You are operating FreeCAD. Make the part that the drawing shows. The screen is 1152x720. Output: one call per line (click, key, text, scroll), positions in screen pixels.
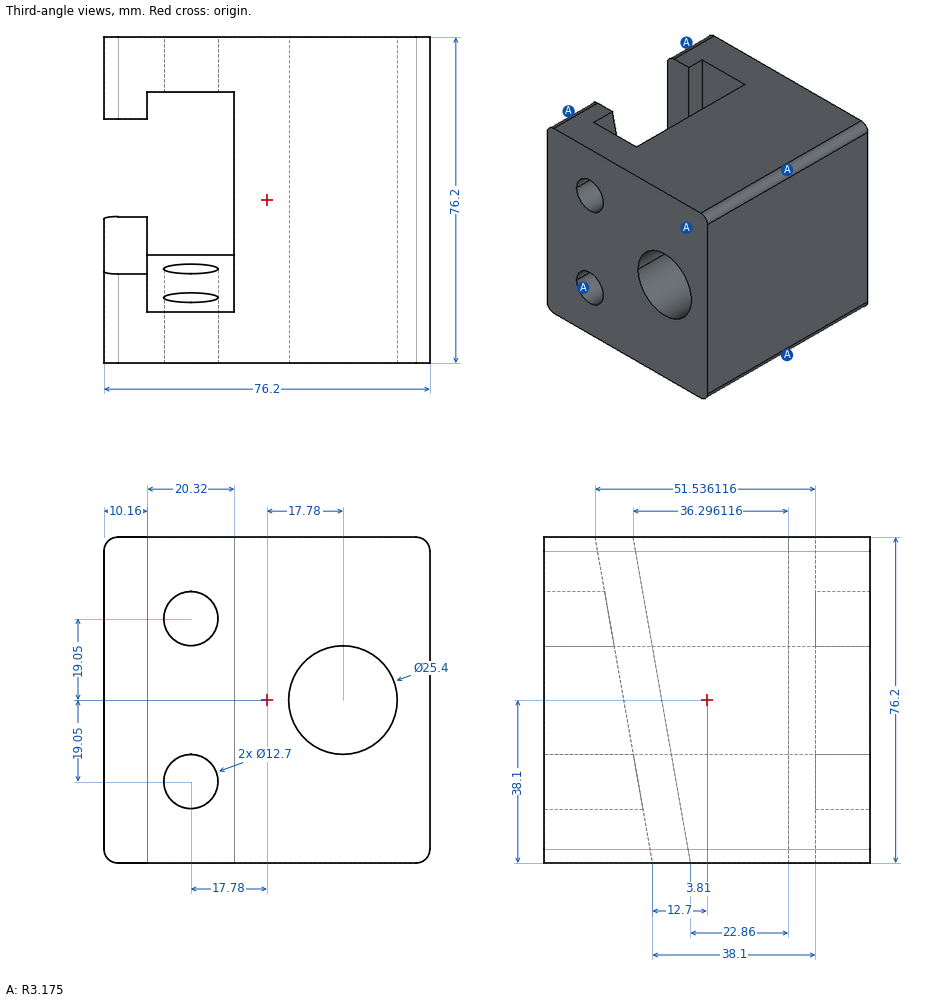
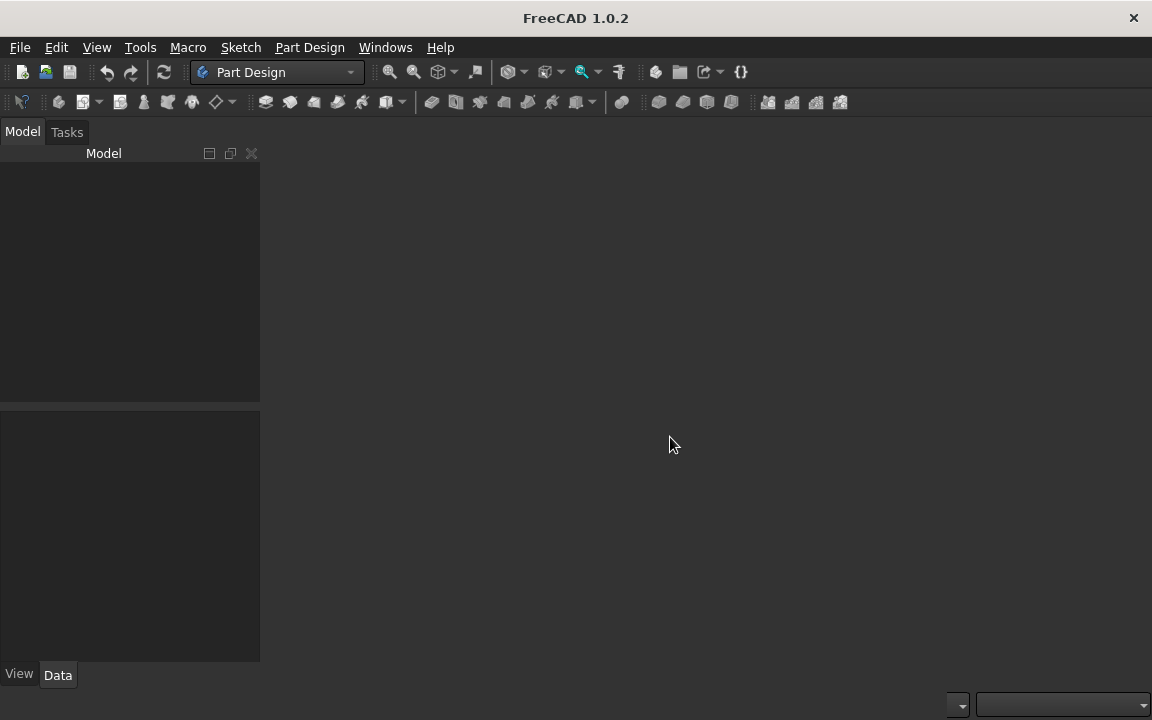
key(ctrl+n)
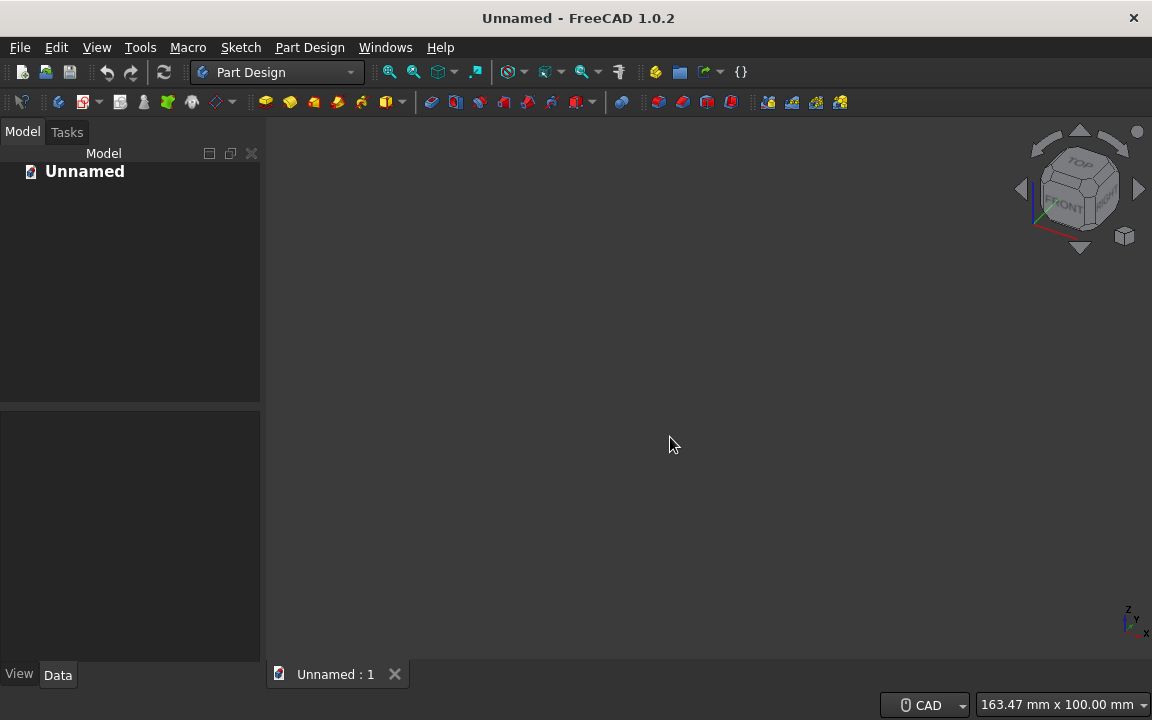
click(84, 102)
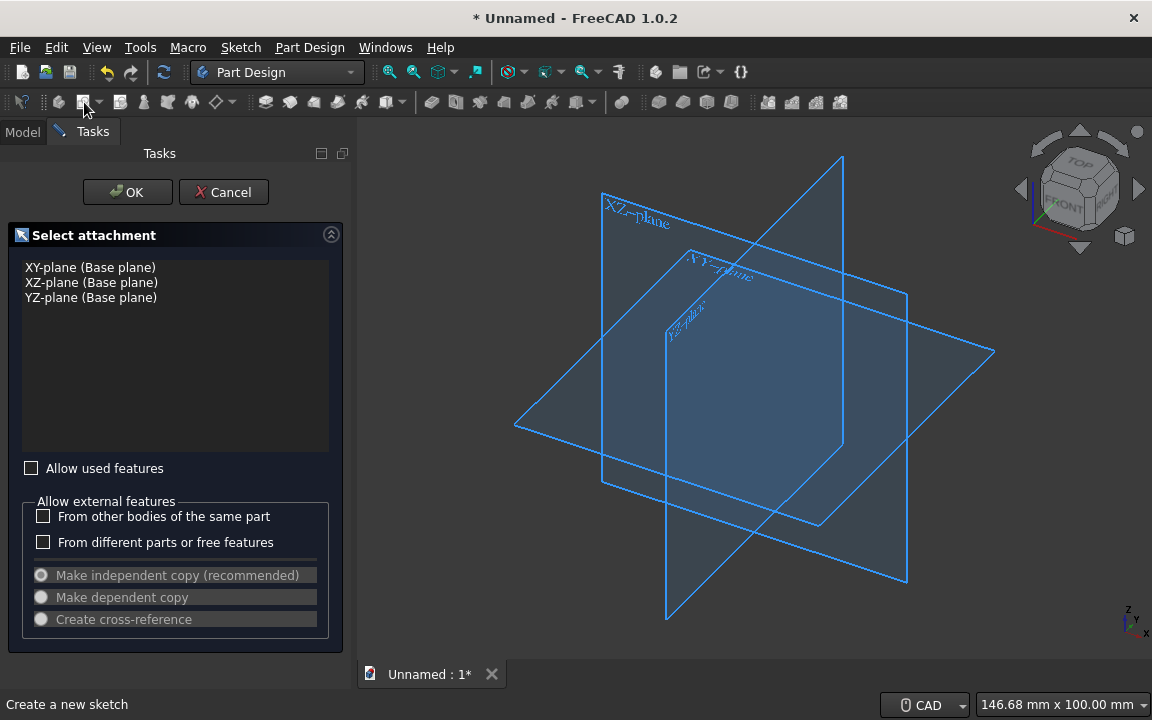
click(82, 268)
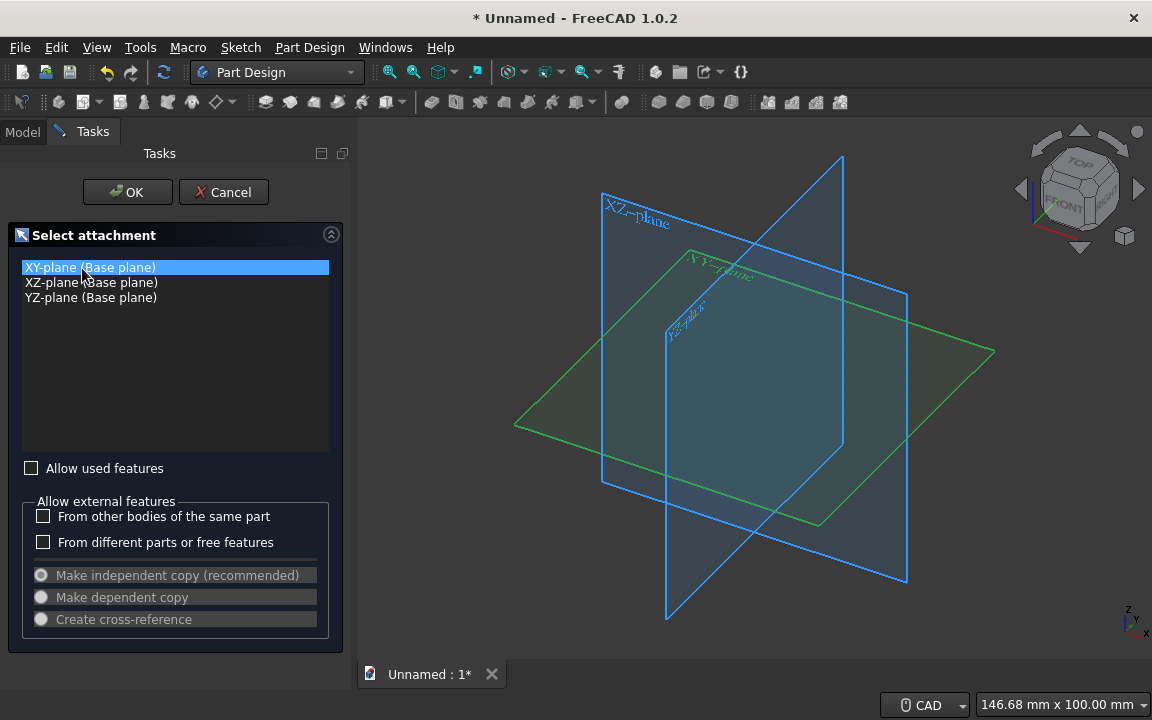
click(128, 192)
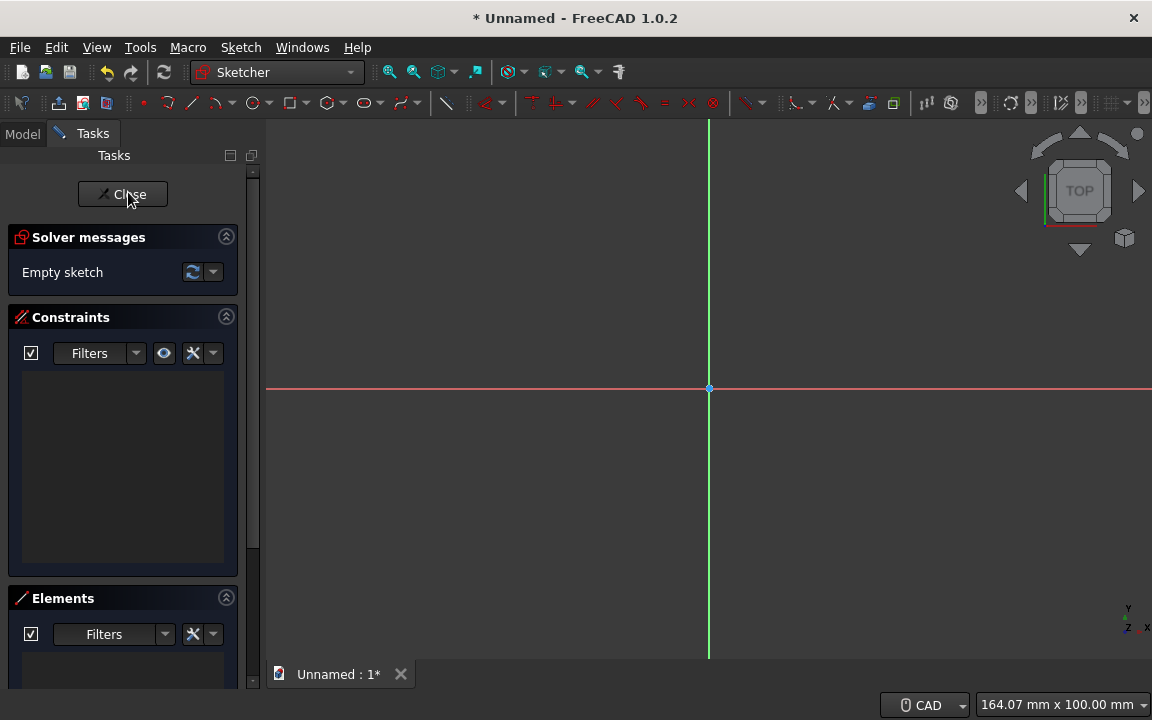
key(g)
key(v)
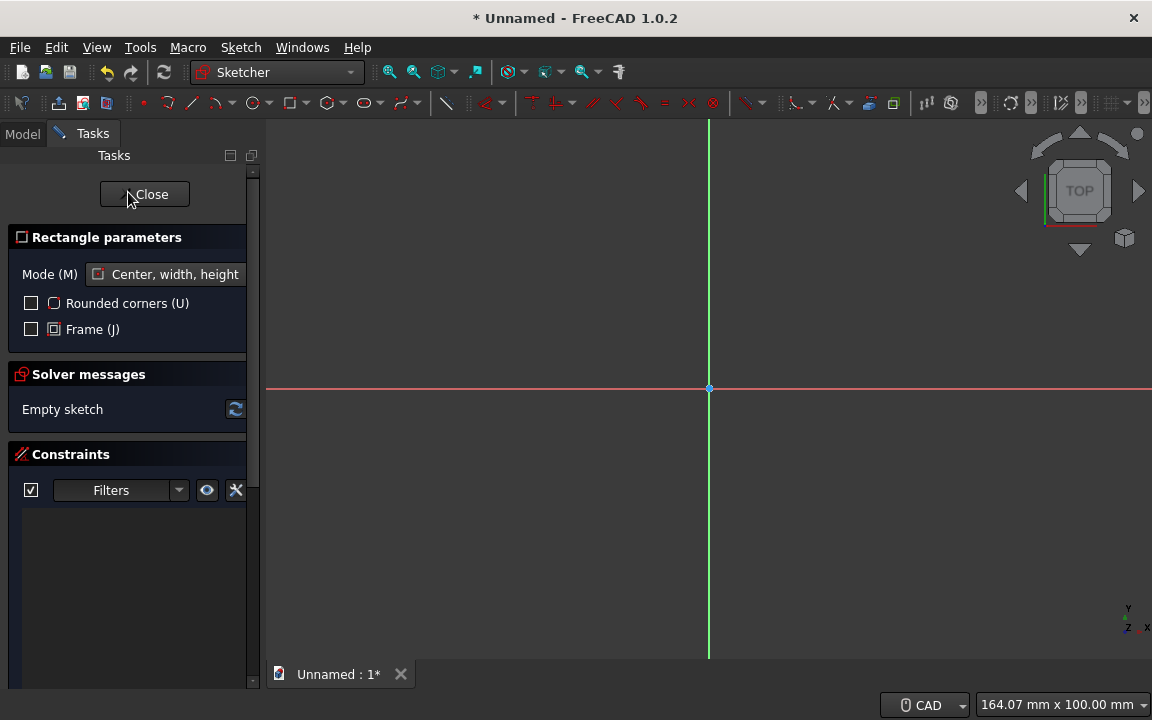
click(709, 389)
click(915, 183)
key(Escape)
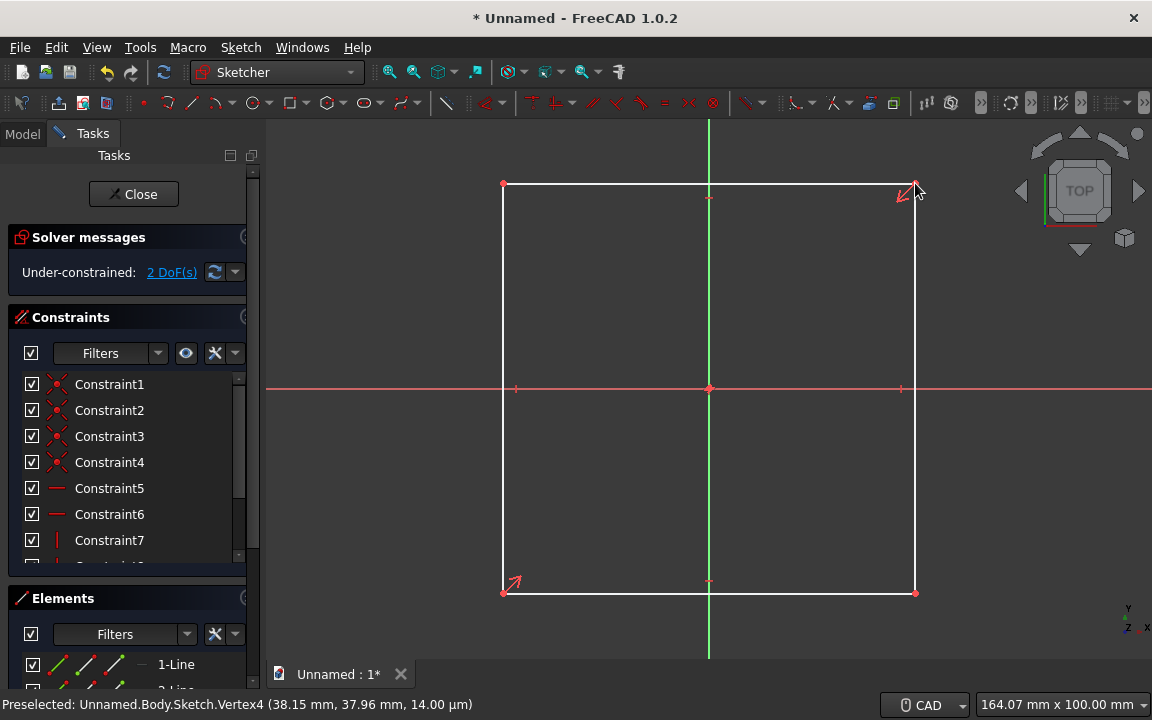
key(d)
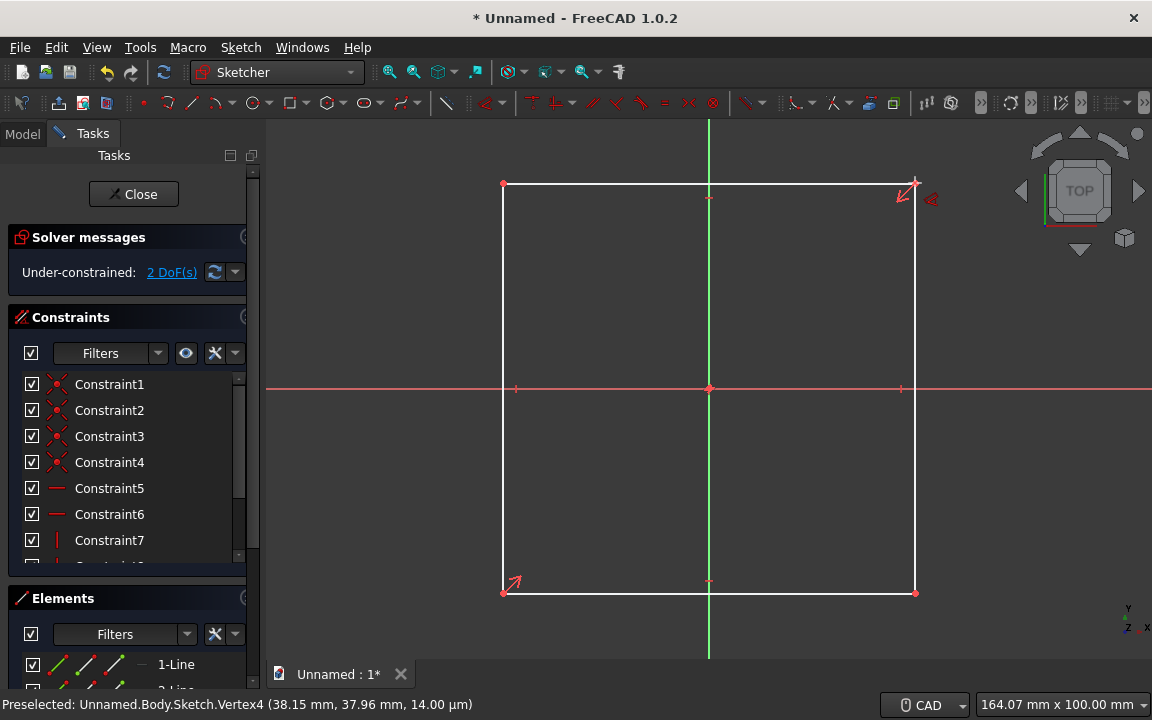
click(627, 594)
click(614, 628)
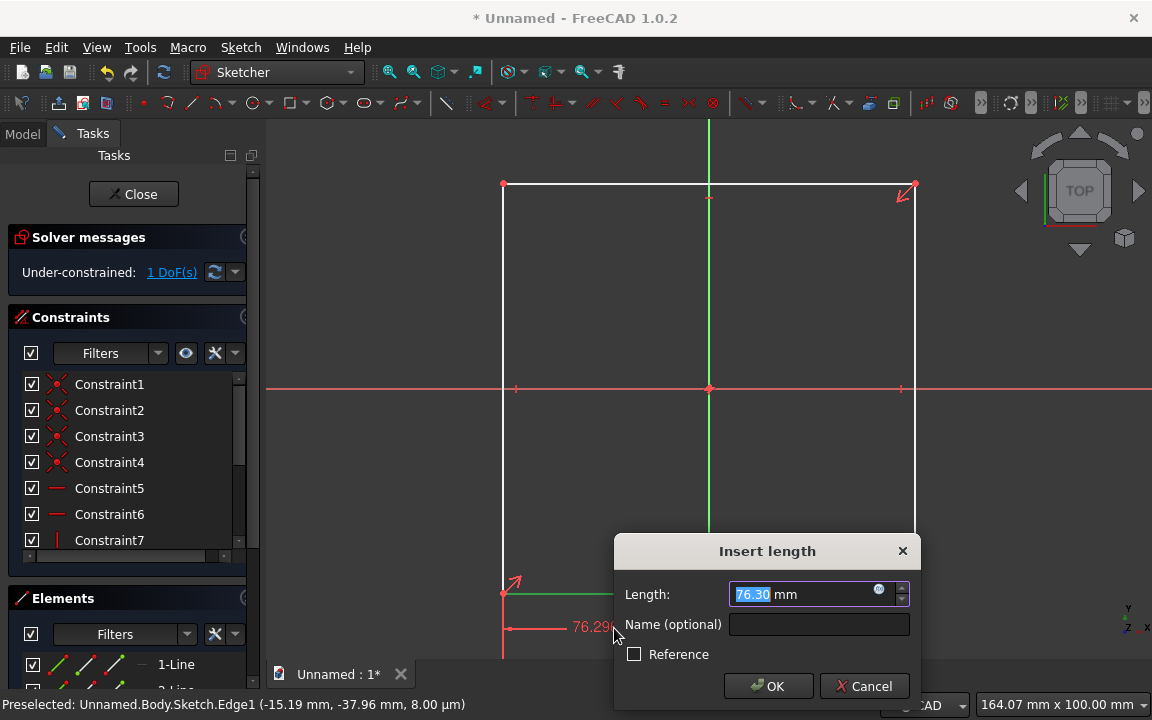
text(76.2)
key(Return)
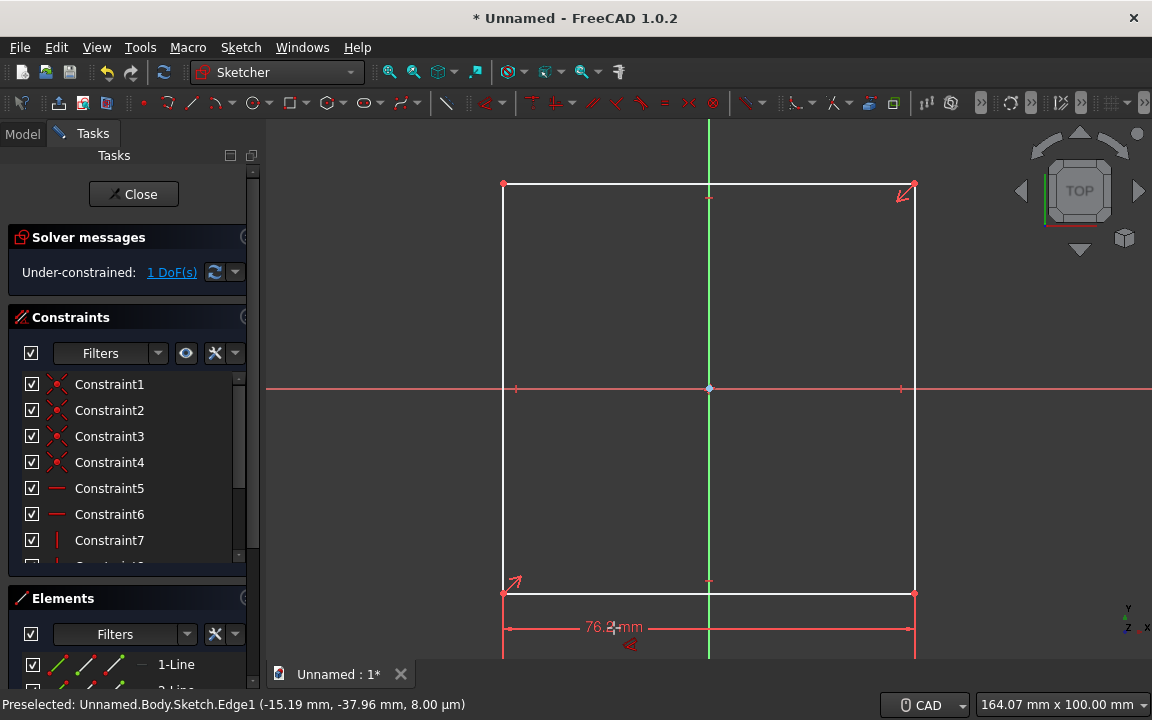
click(915, 471)
click(949, 295)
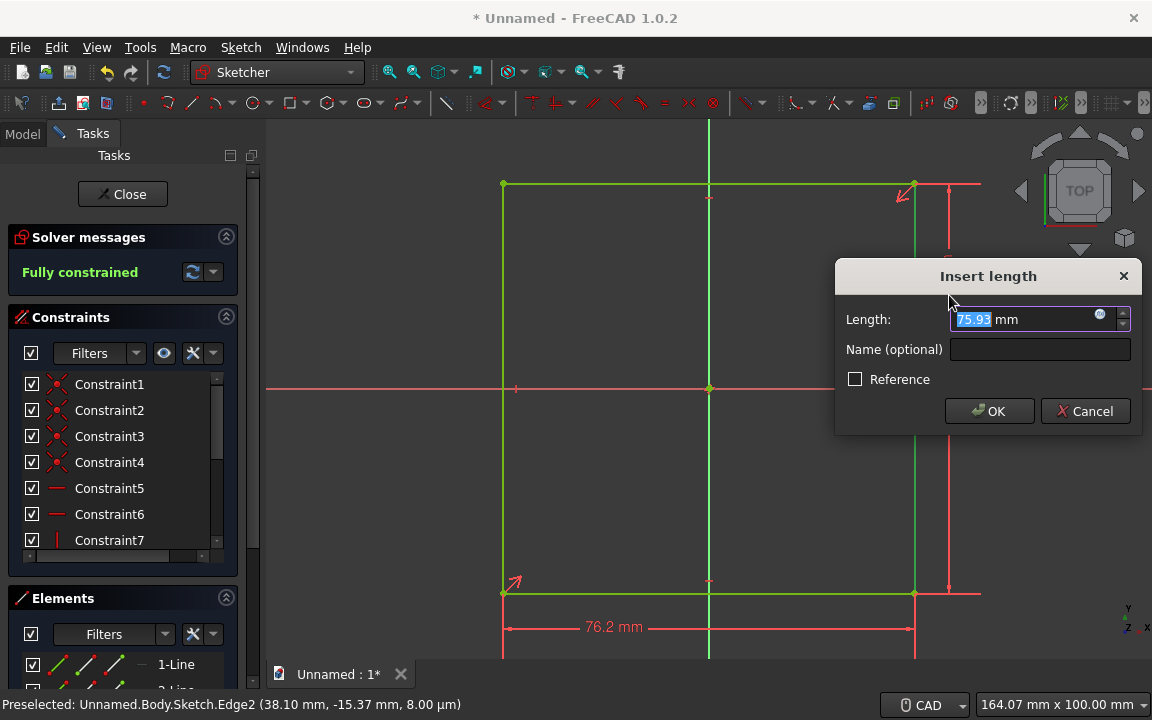
text(76.2)
key(Return)
key(Escape)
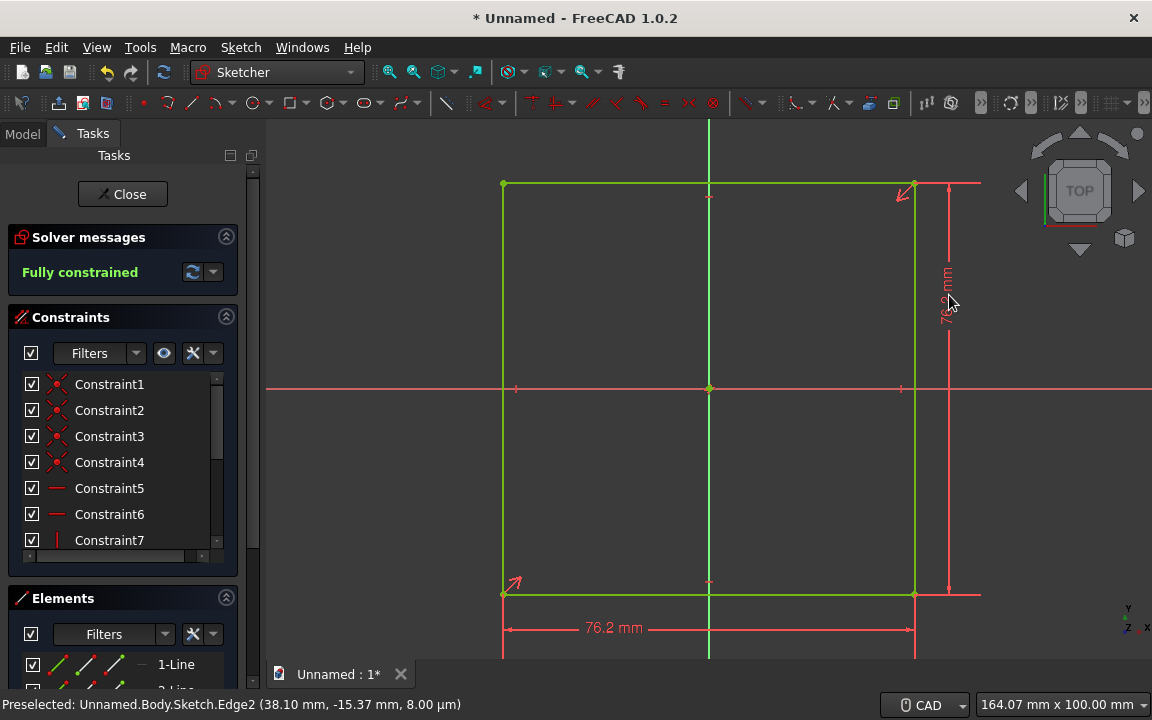
click(123, 194)